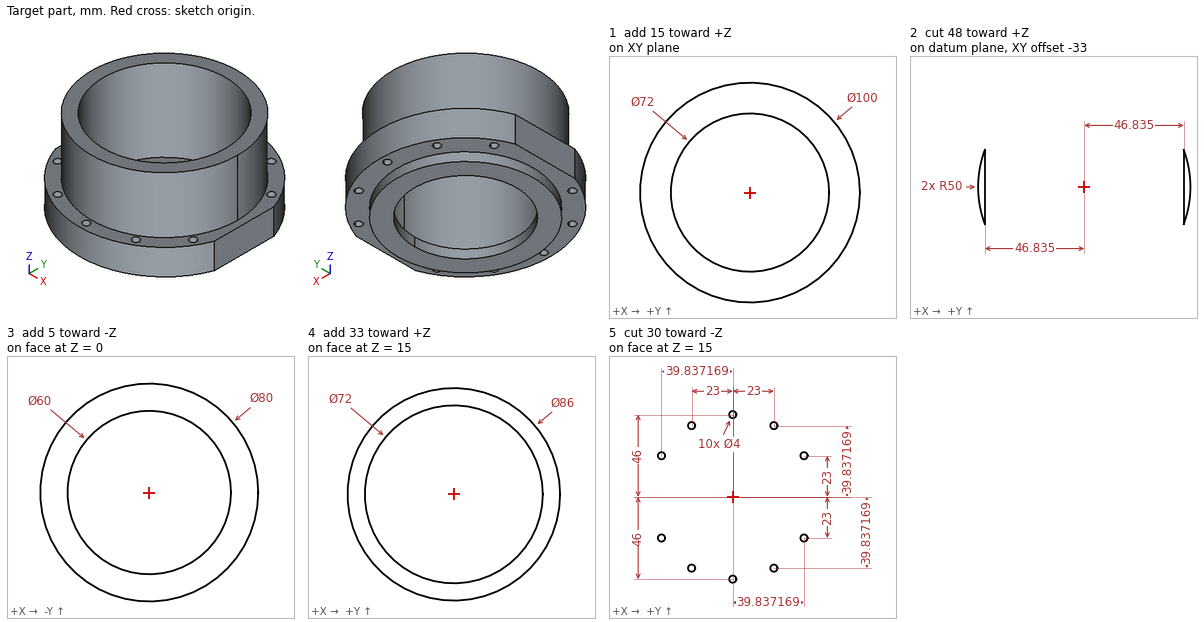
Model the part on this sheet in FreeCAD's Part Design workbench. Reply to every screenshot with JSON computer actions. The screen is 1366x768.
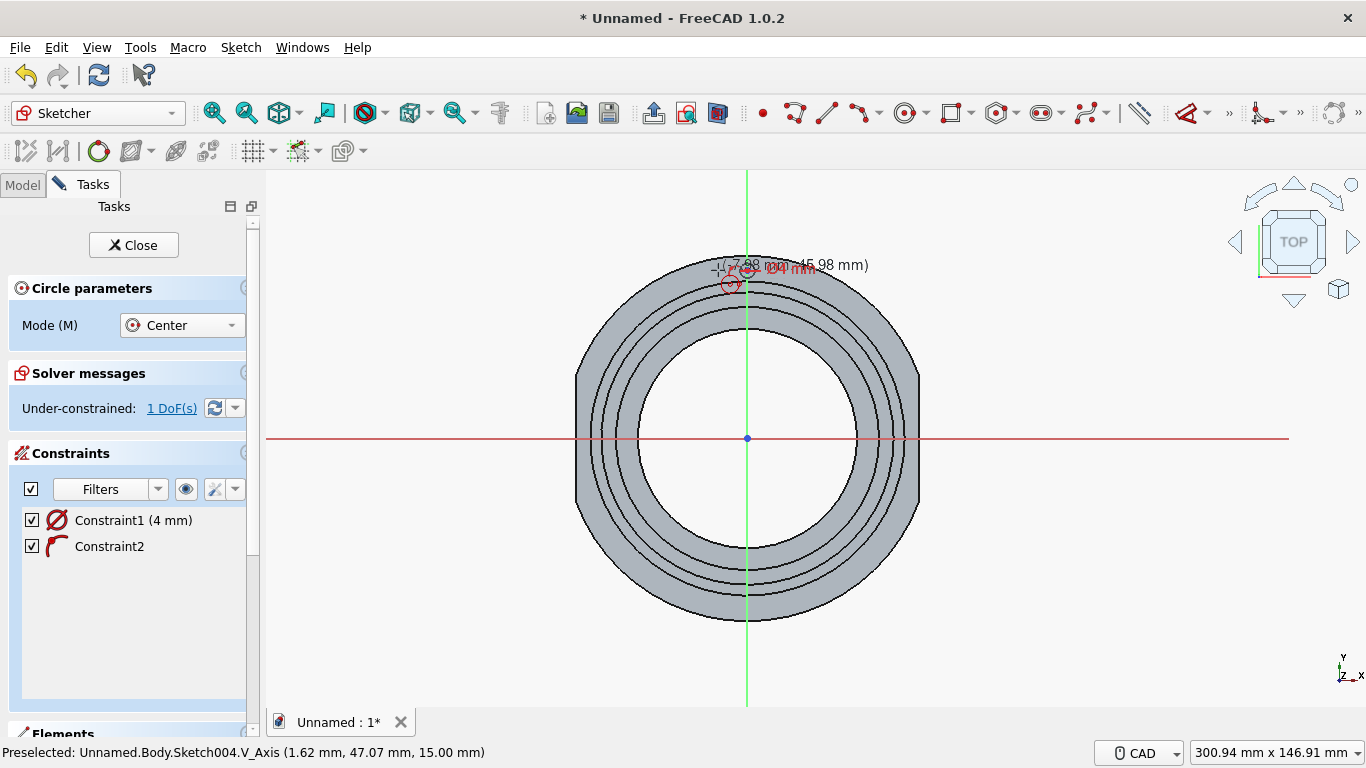
{"action": "scroll", "coordinate": [893, 523], "scroll_direction": "up", "scroll_amount": 6}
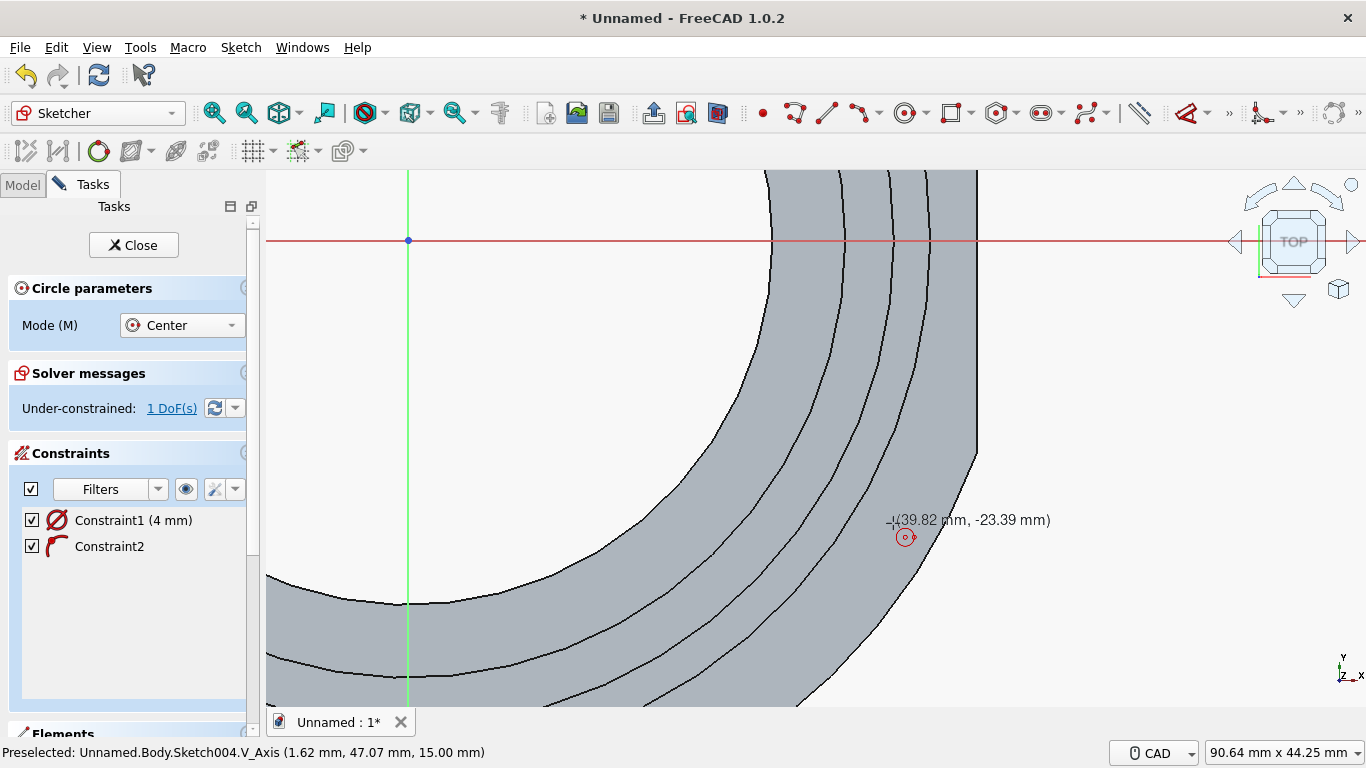
{"action": "left_click", "coordinate": [892, 520]}
{"action": "mouse_move", "coordinate": [909, 503]}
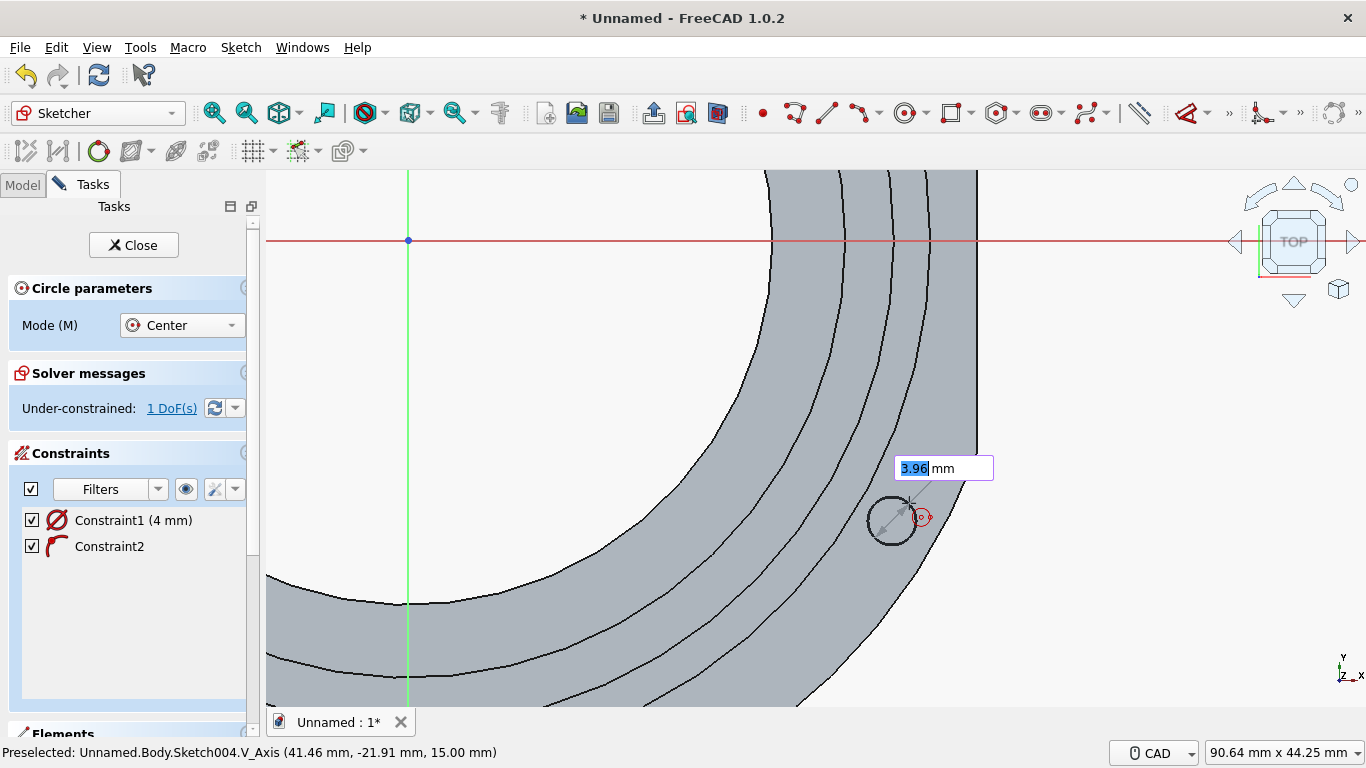
{"action": "type", "text": "4"}
{"action": "key", "text": "Return"}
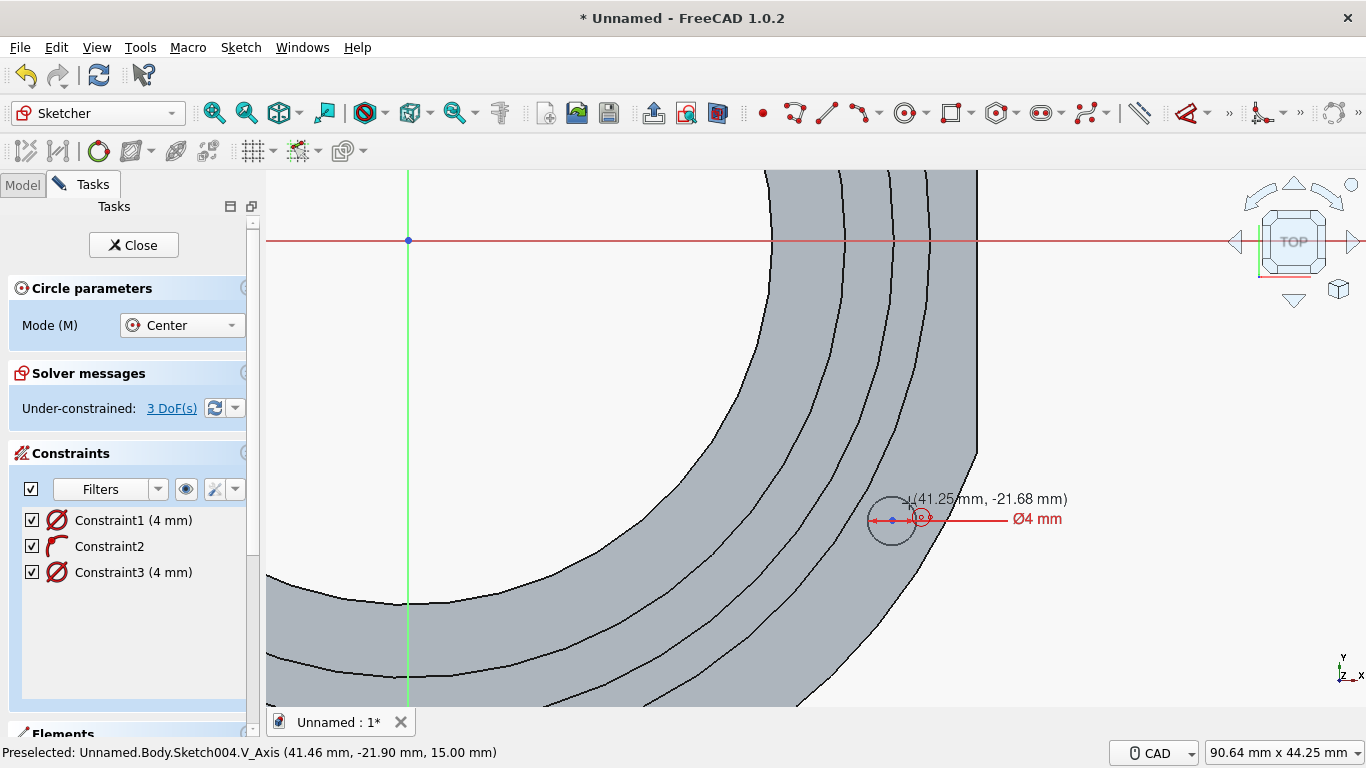
{"action": "scroll", "coordinate": [894, 524], "scroll_direction": "down", "scroll_amount": 6}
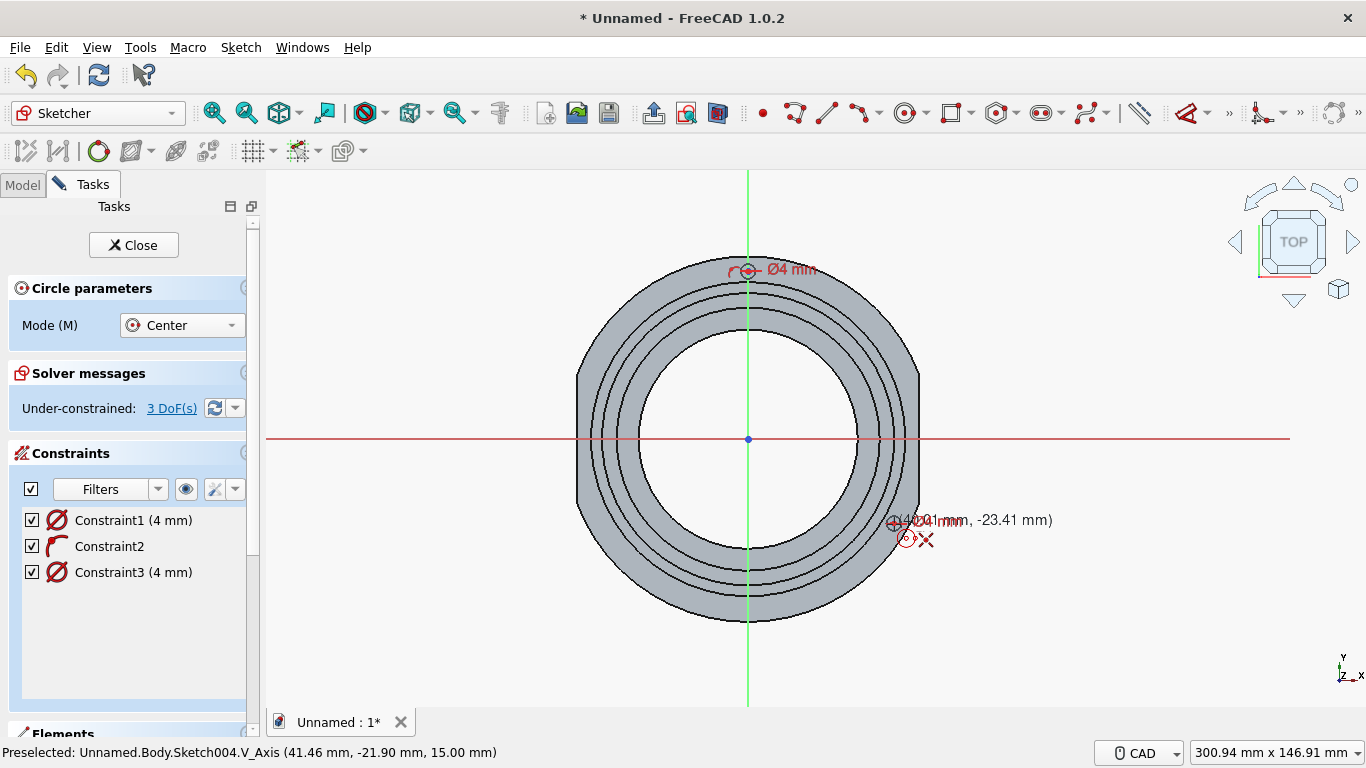
{"action": "scroll", "coordinate": [832, 294], "scroll_direction": "up", "scroll_amount": 6}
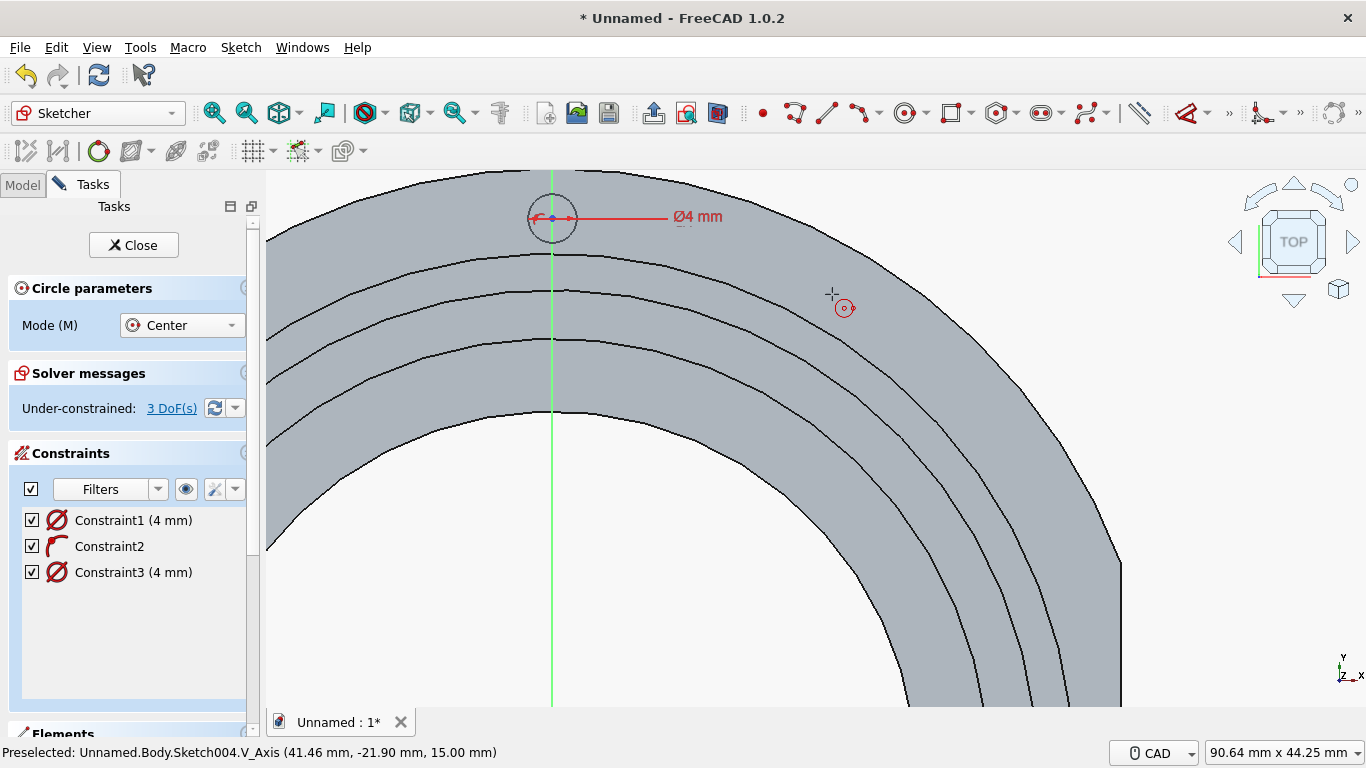
{"action": "left_click", "coordinate": [832, 292]}
{"action": "mouse_move", "coordinate": [849, 275]}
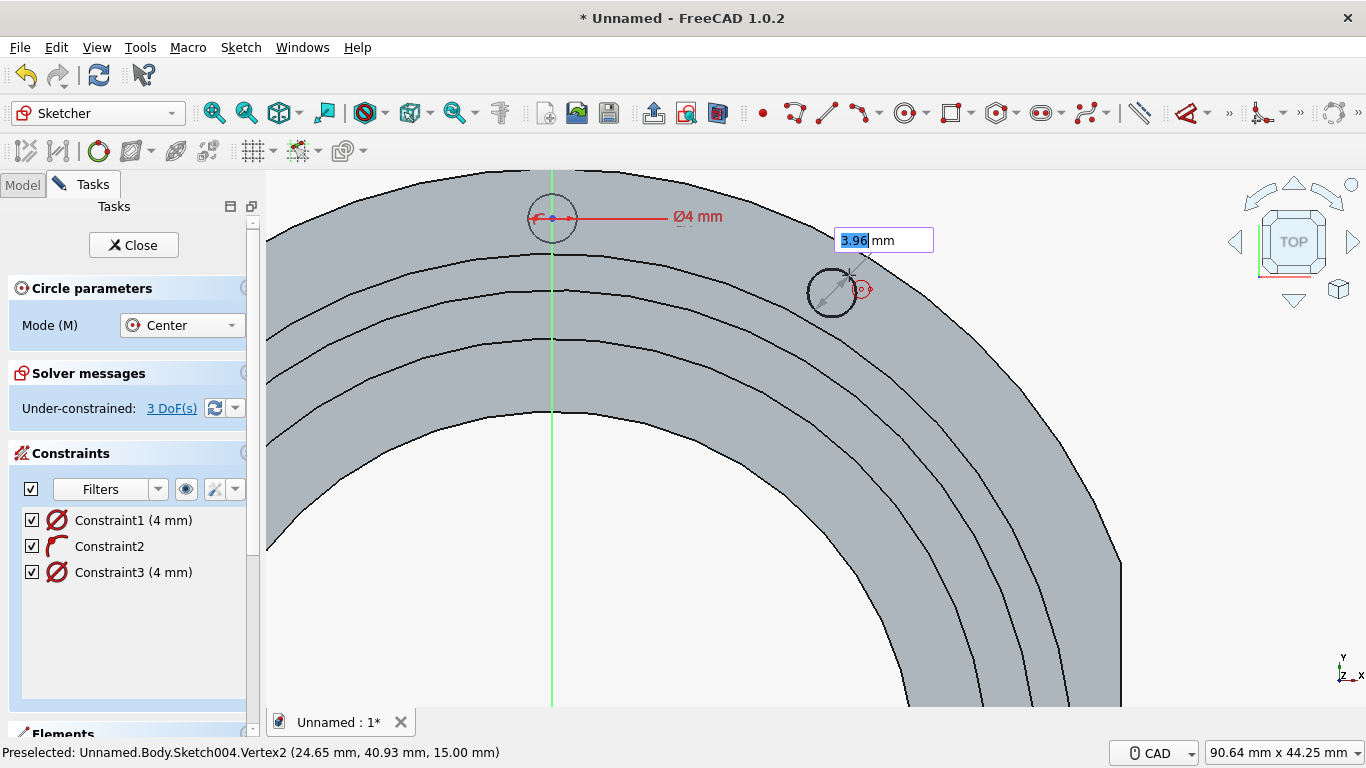
{"action": "type", "text": "4"}
{"action": "key", "text": "Return"}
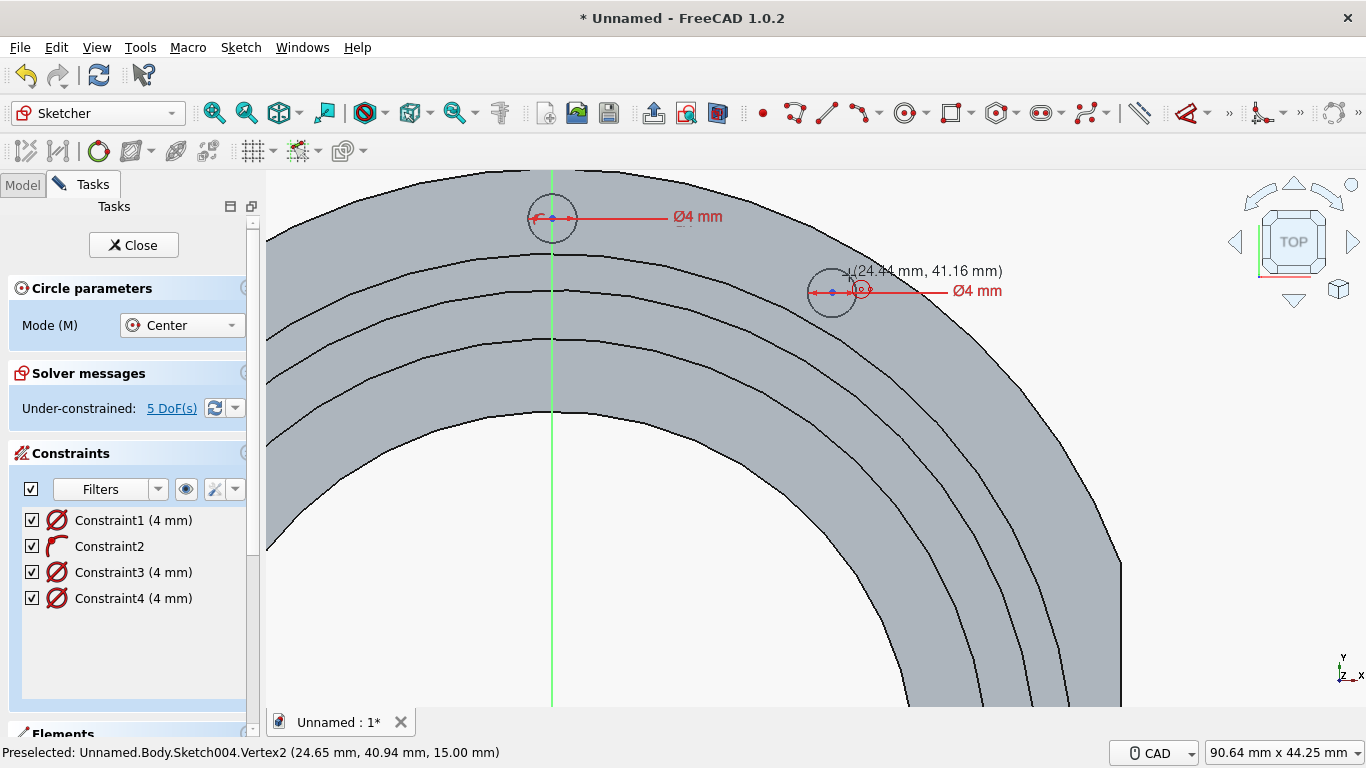
{"action": "left_click", "coordinate": [1036, 496]}
{"action": "mouse_move", "coordinate": [1053, 479]}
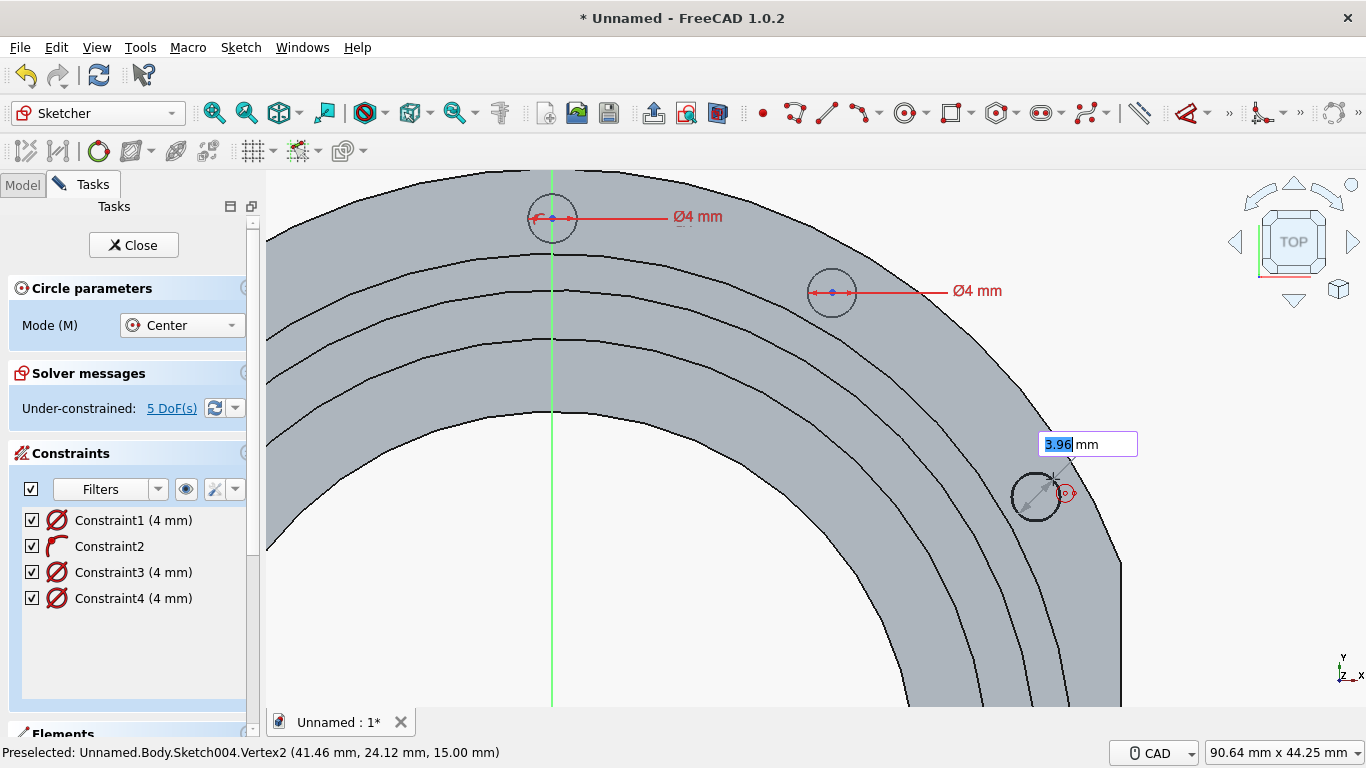
{"action": "type", "text": "4"}
{"action": "key", "text": "Return"}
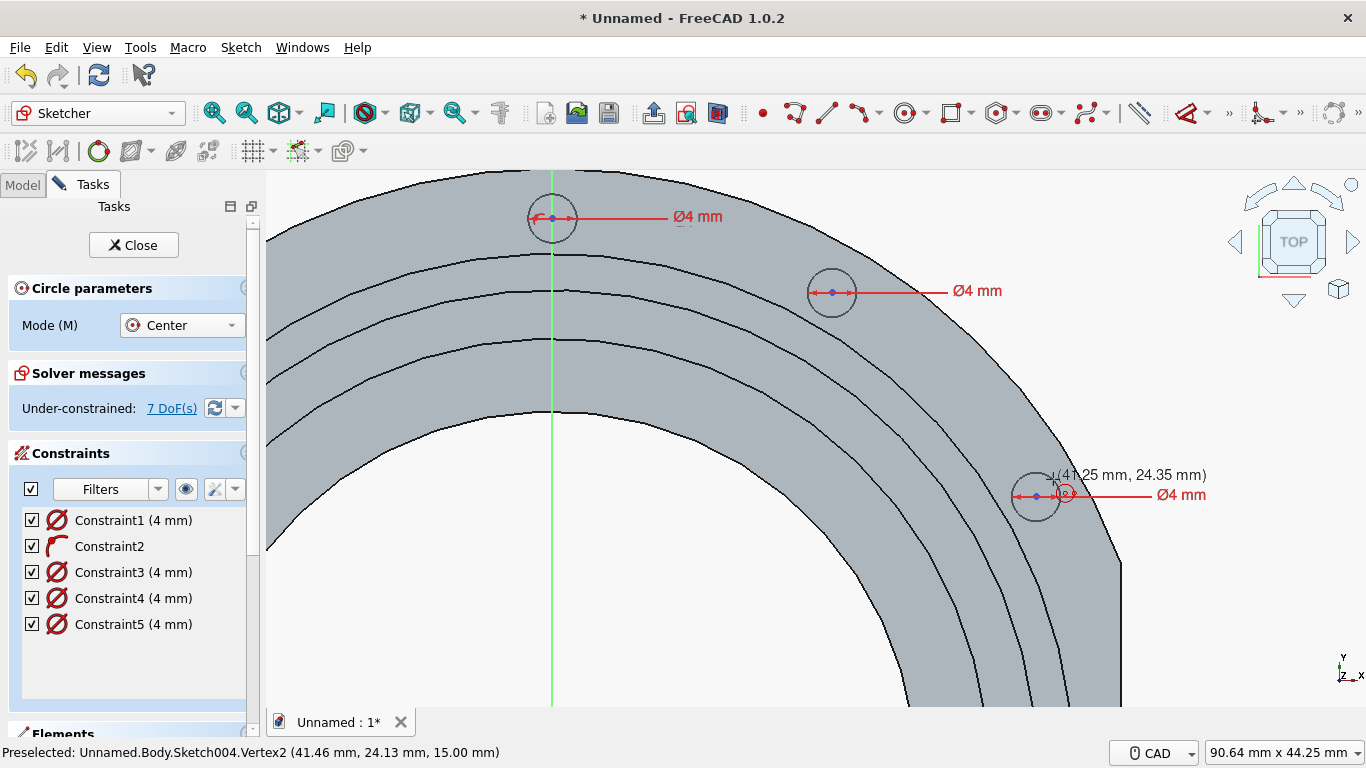
{"action": "scroll", "coordinate": [832, 293], "scroll_direction": "down", "scroll_amount": 6}